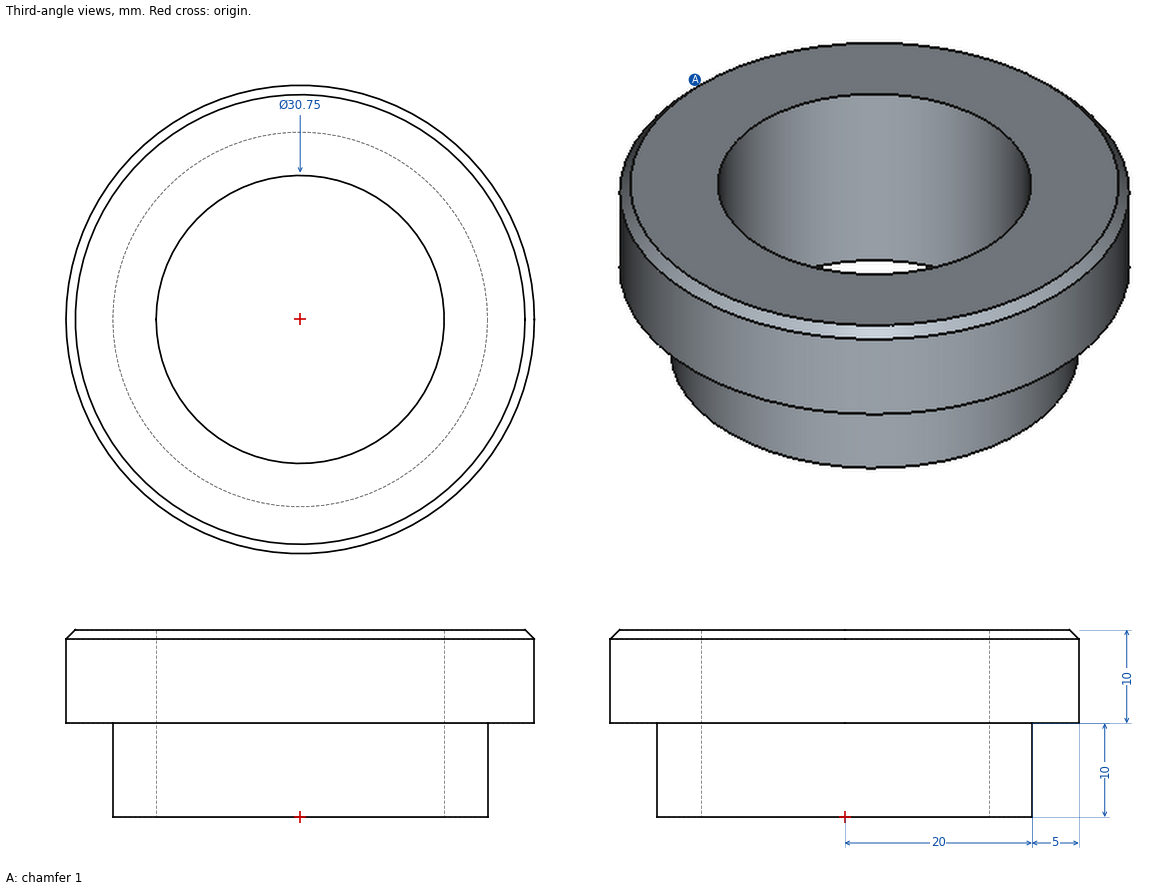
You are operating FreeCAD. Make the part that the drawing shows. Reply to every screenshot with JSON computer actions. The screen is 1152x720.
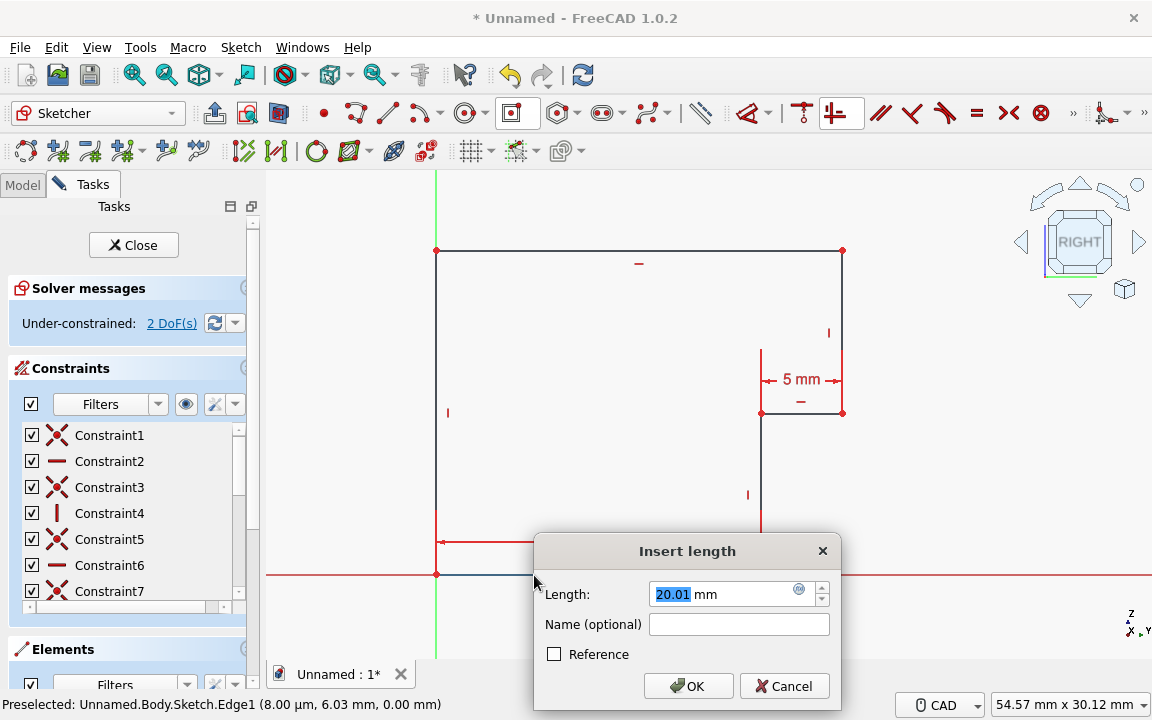
{"action": "type", "text": "20"}
{"action": "key", "text": "Return"}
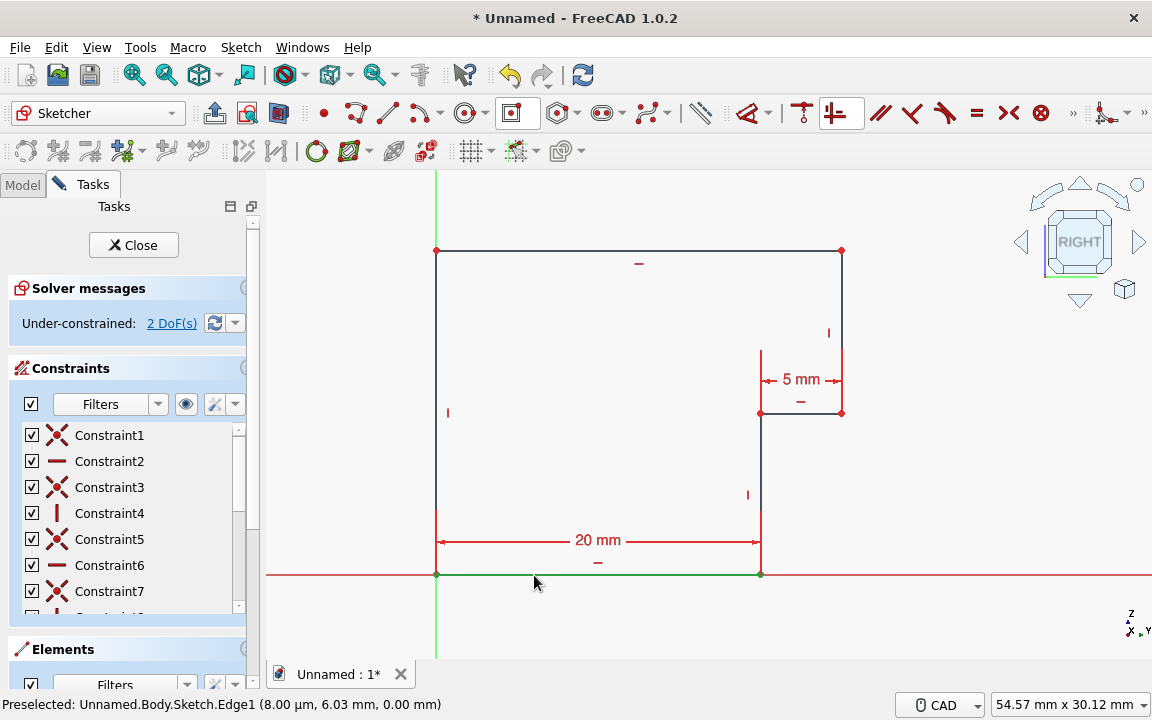
{"action": "left_click", "coordinate": [761, 527]}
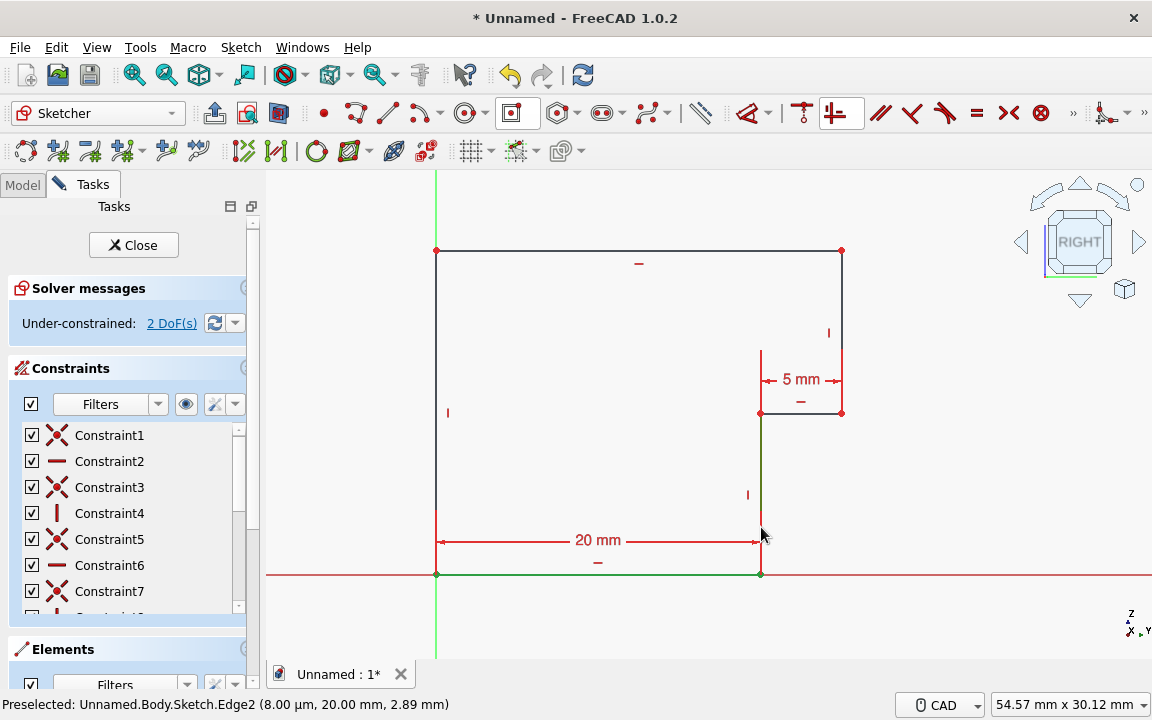
{"action": "key", "text": "i"}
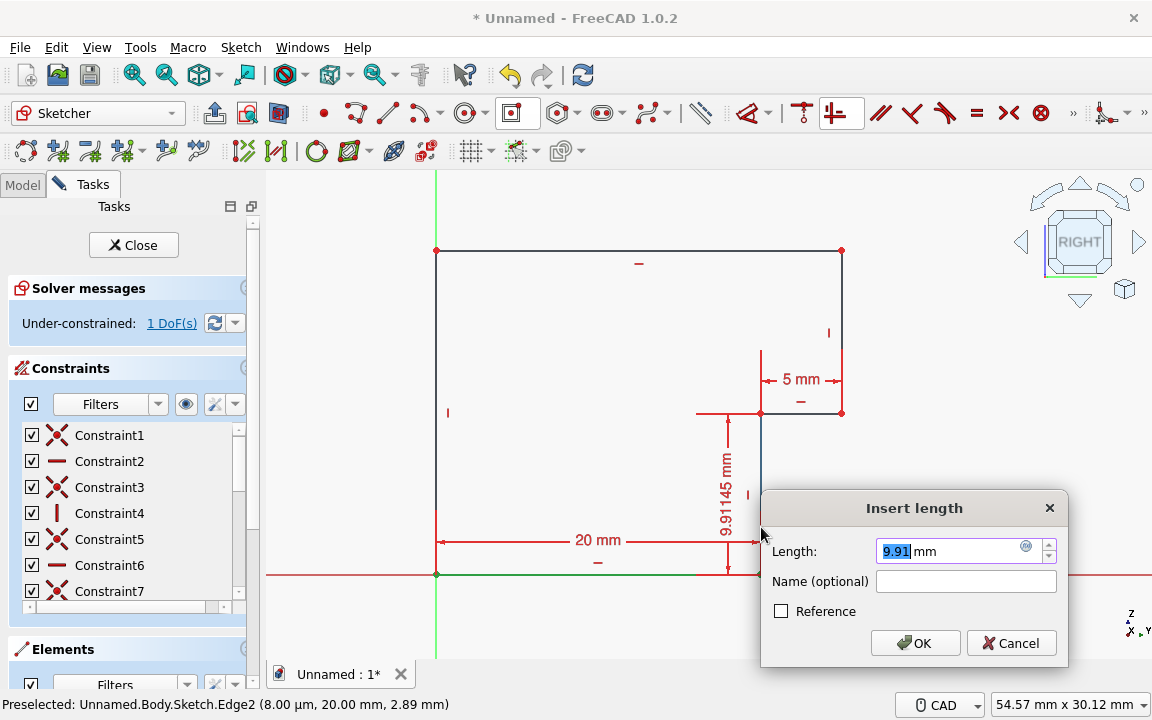
{"action": "type", "text": "10"}
{"action": "key", "text": "Return"}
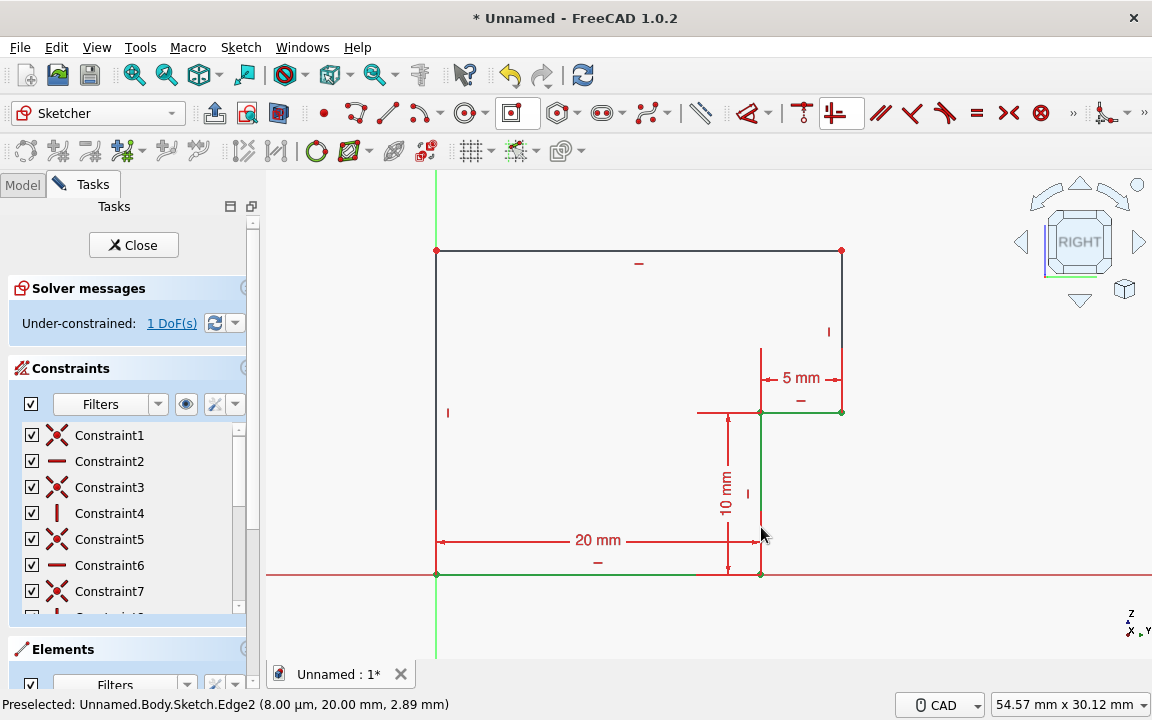
{"action": "left_click", "coordinate": [842, 364]}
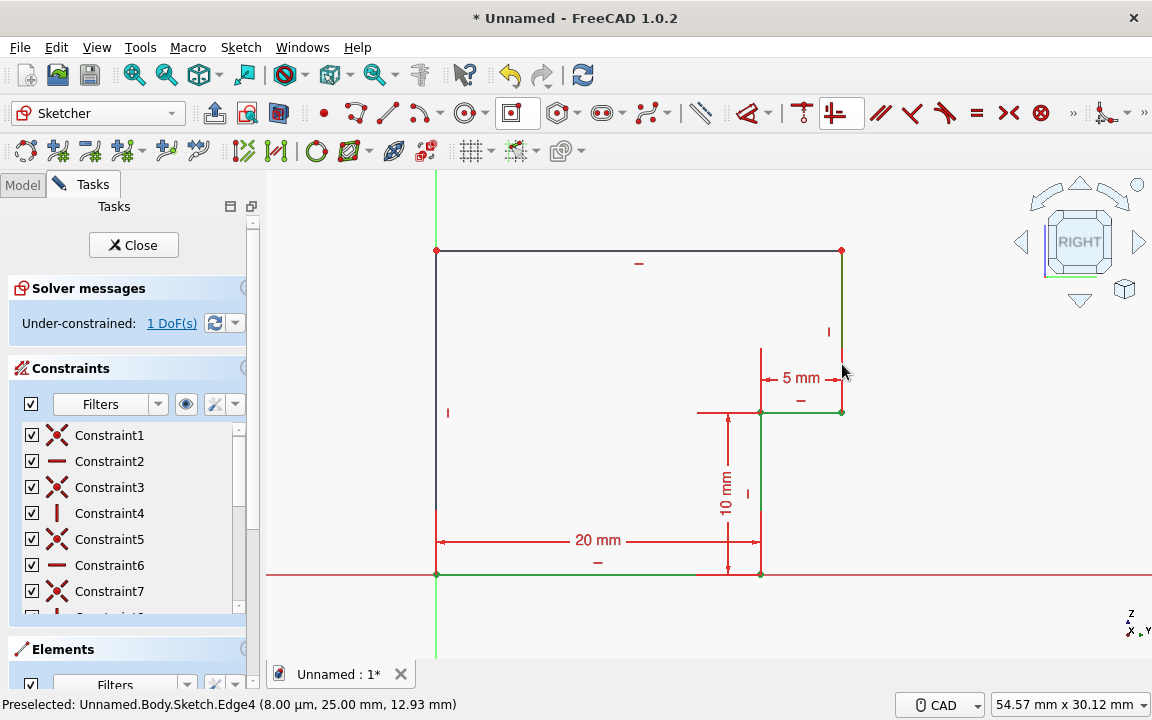
{"action": "key", "text": "i"}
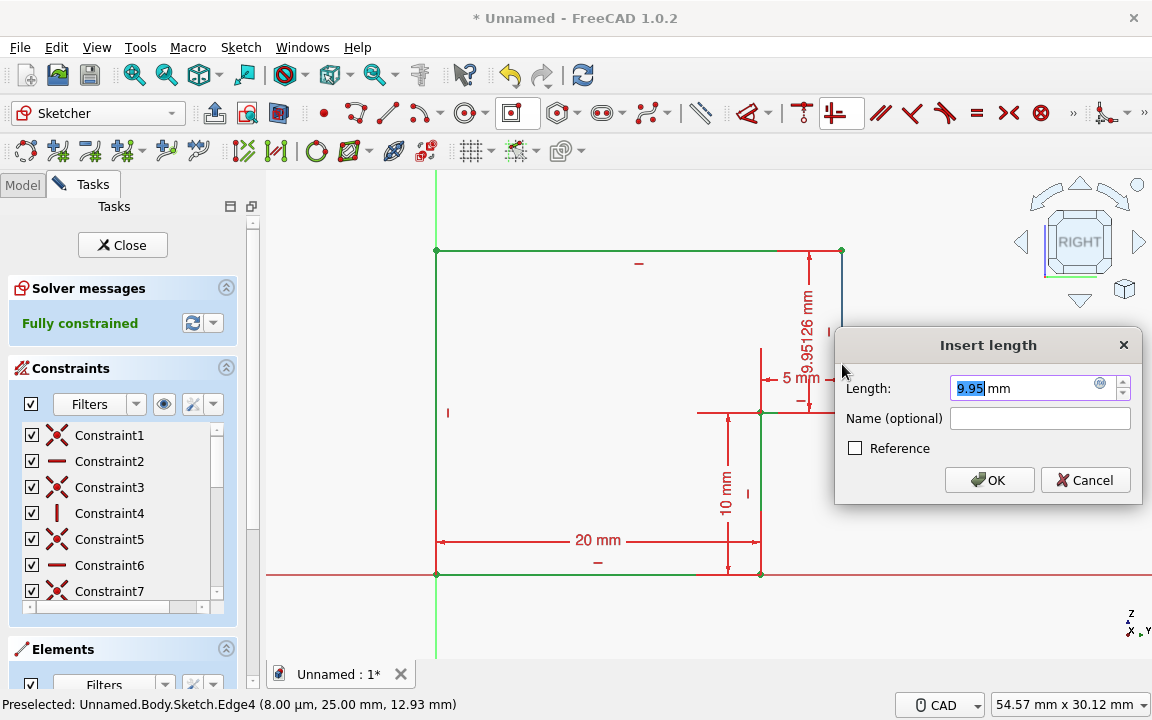
{"action": "type", "text": "10"}
{"action": "key", "text": "Return"}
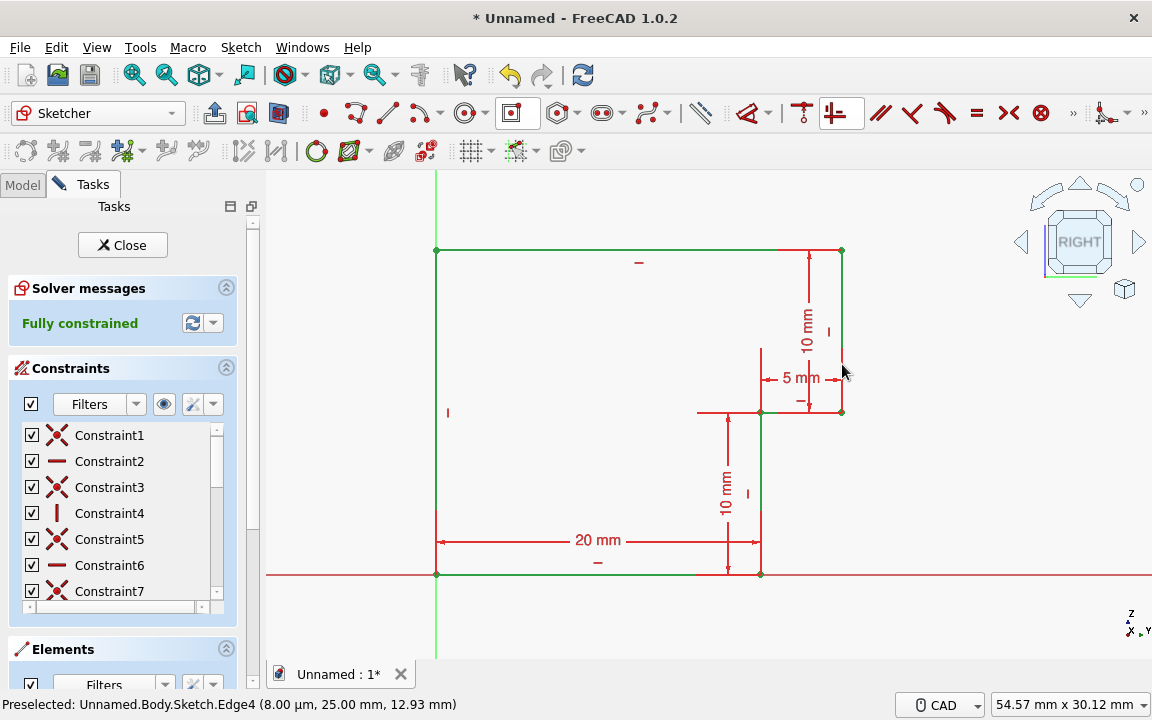
{"action": "left_click", "coordinate": [123, 245]}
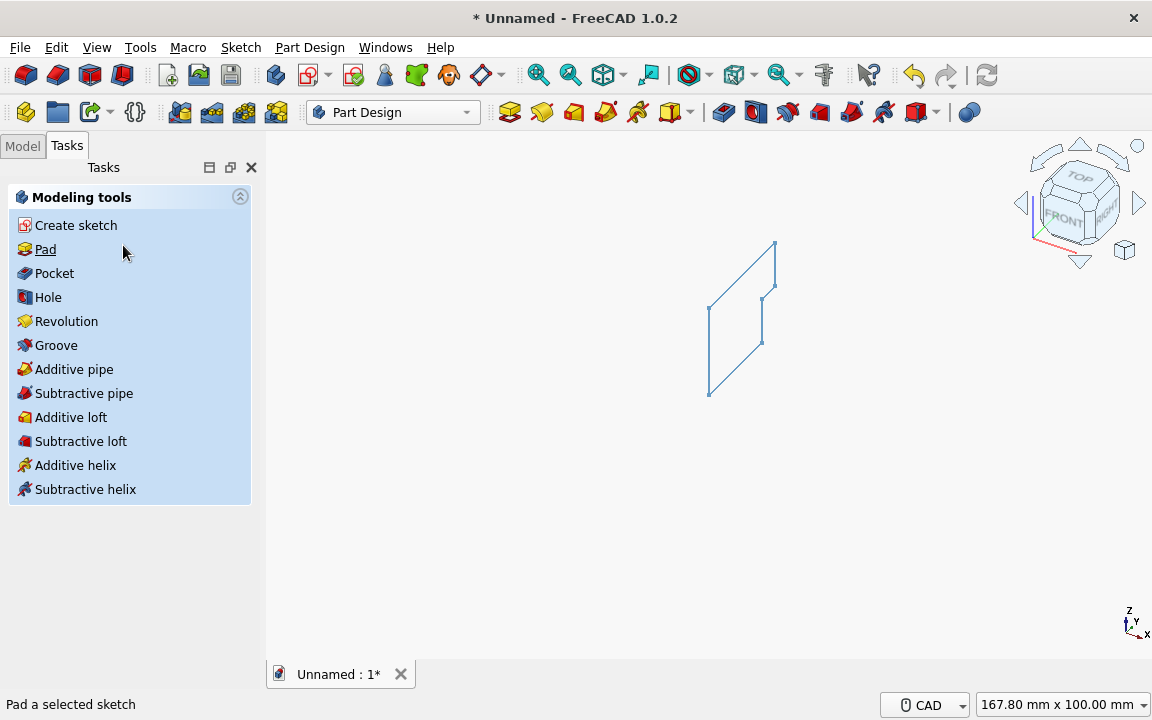
{"action": "left_click", "coordinate": [542, 112]}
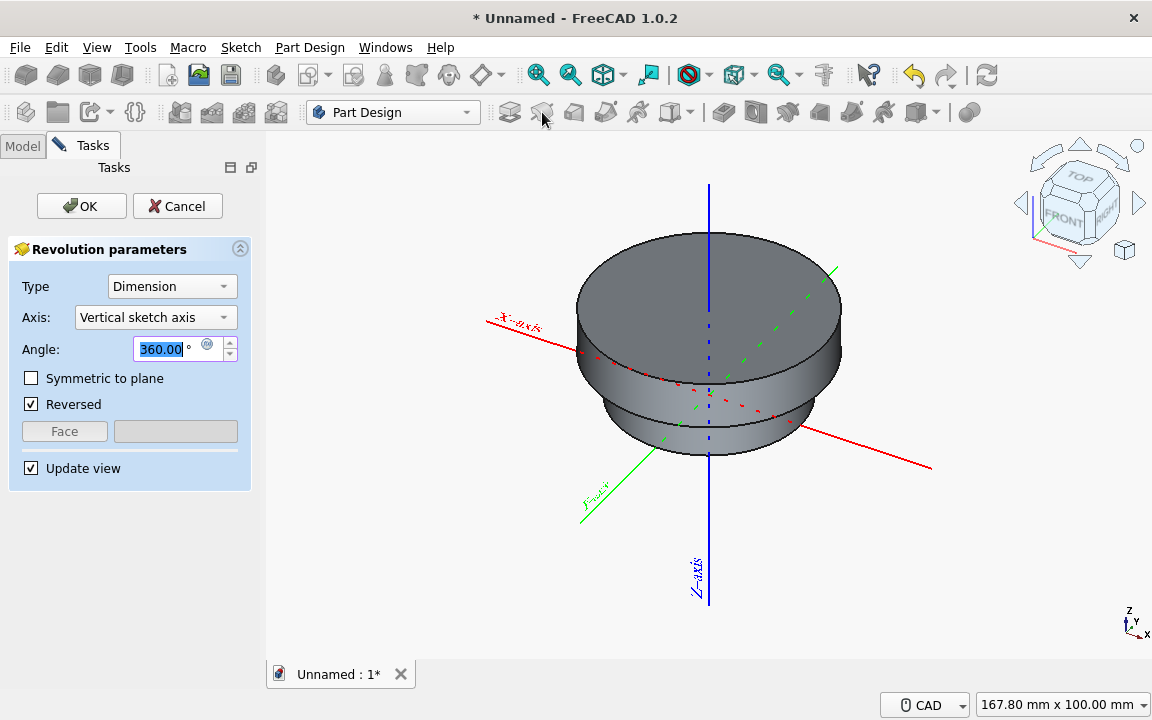
{"action": "left_click", "coordinate": [82, 206]}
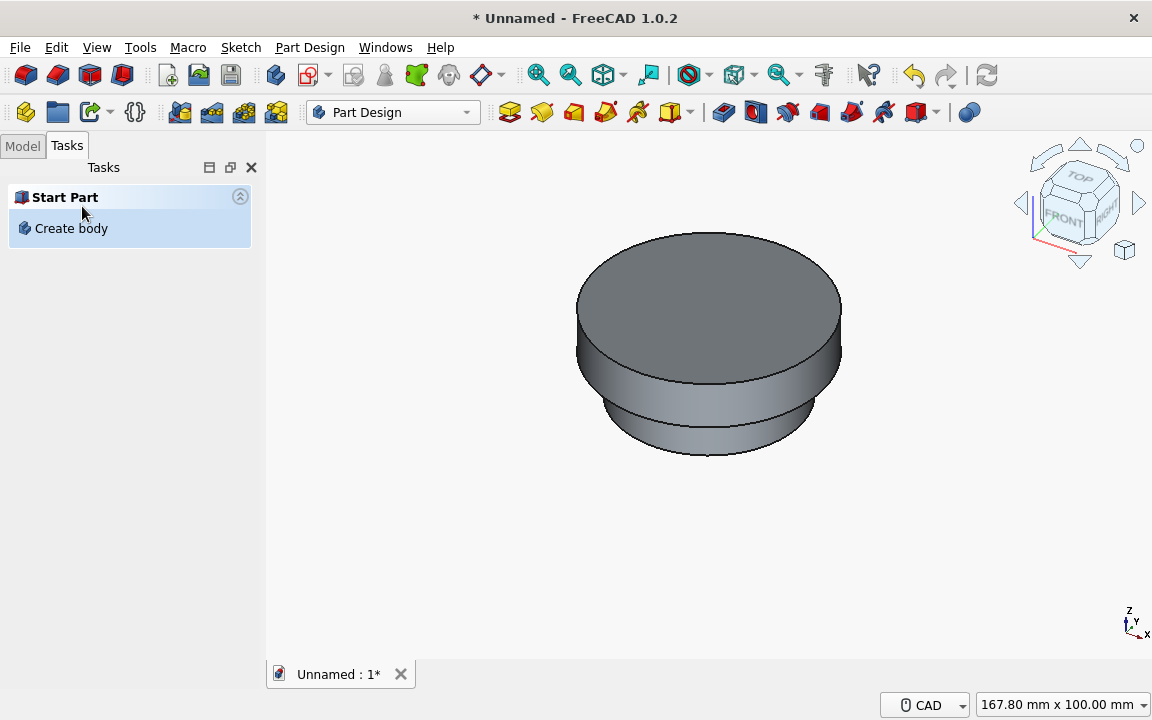
{"action": "left_click", "coordinate": [709, 307]}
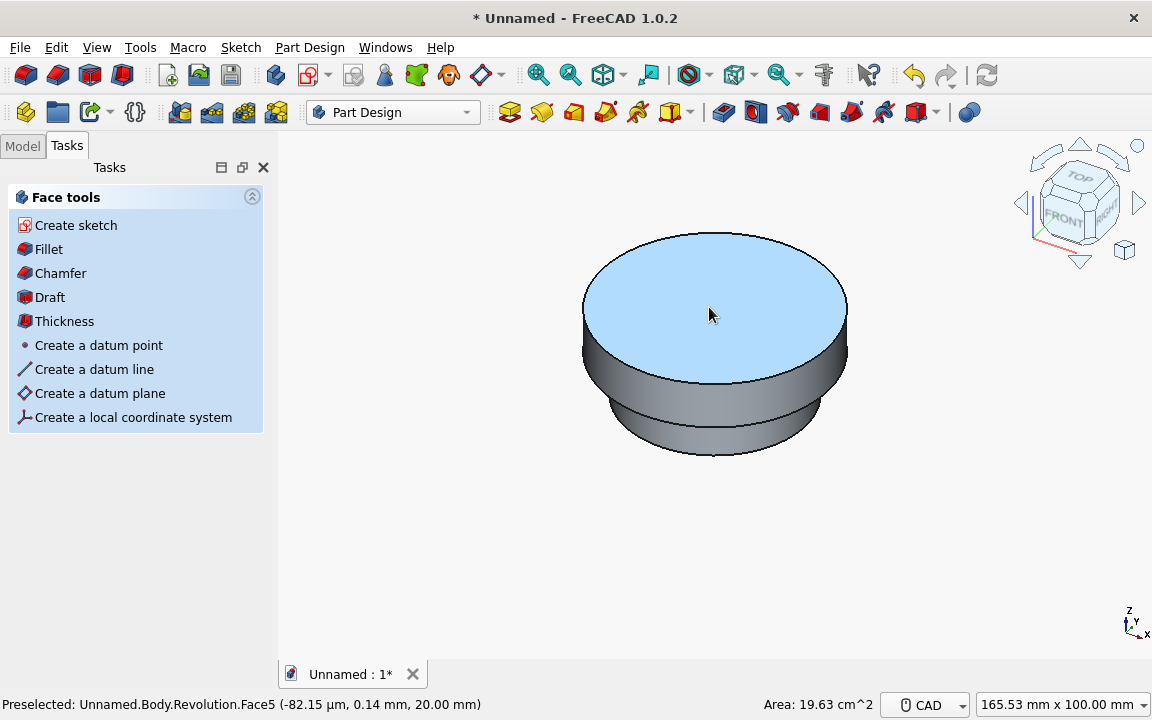
{"action": "left_click", "coordinate": [308, 76]}